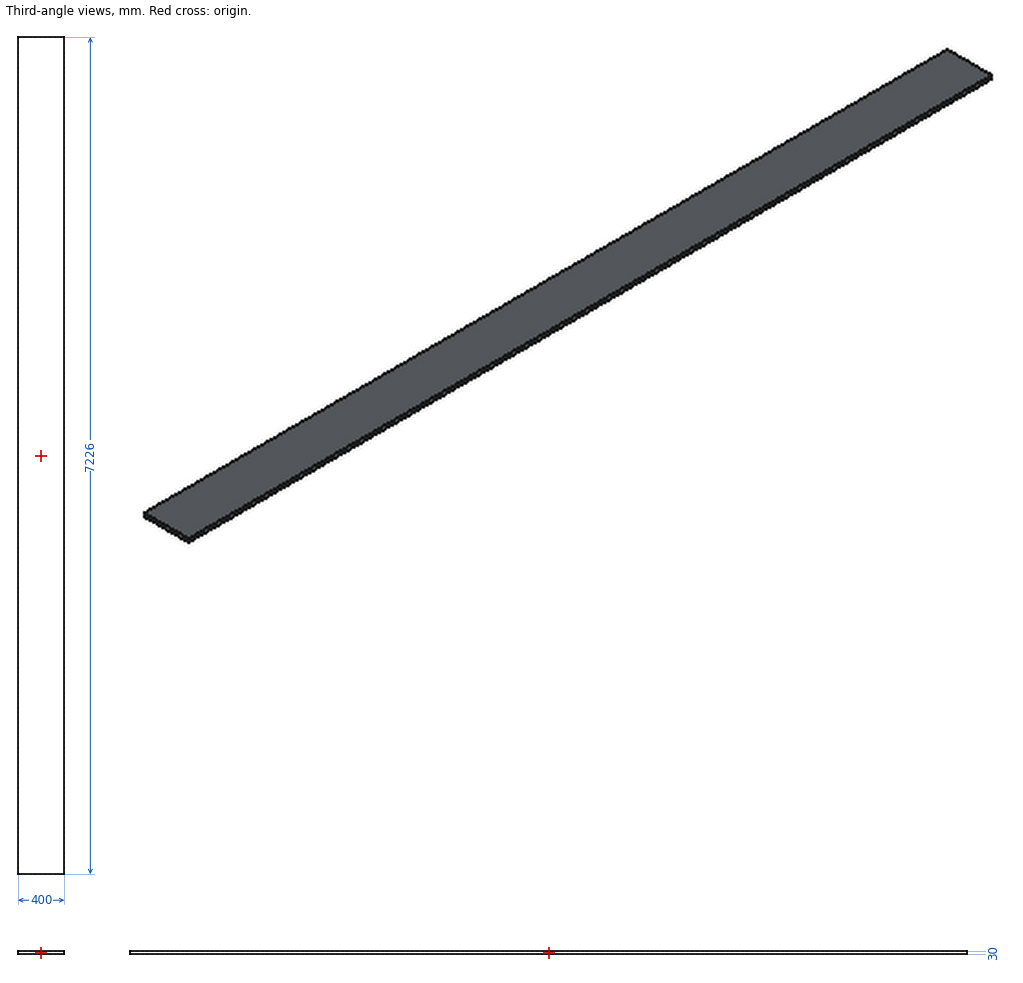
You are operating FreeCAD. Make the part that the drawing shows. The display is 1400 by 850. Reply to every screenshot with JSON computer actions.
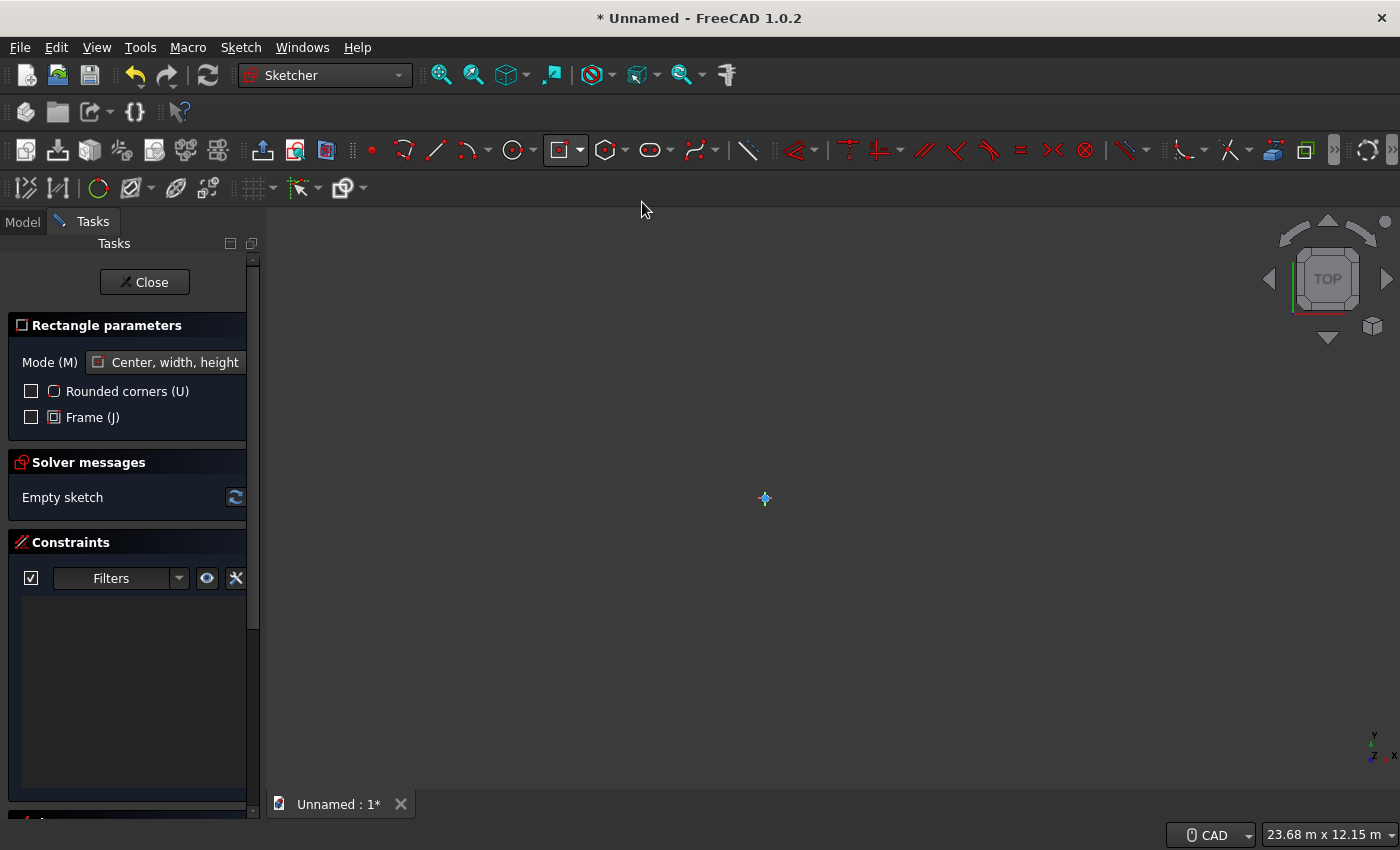
{"action": "scroll", "coordinate": [765, 498], "scroll_direction": "up", "scroll_amount": 3}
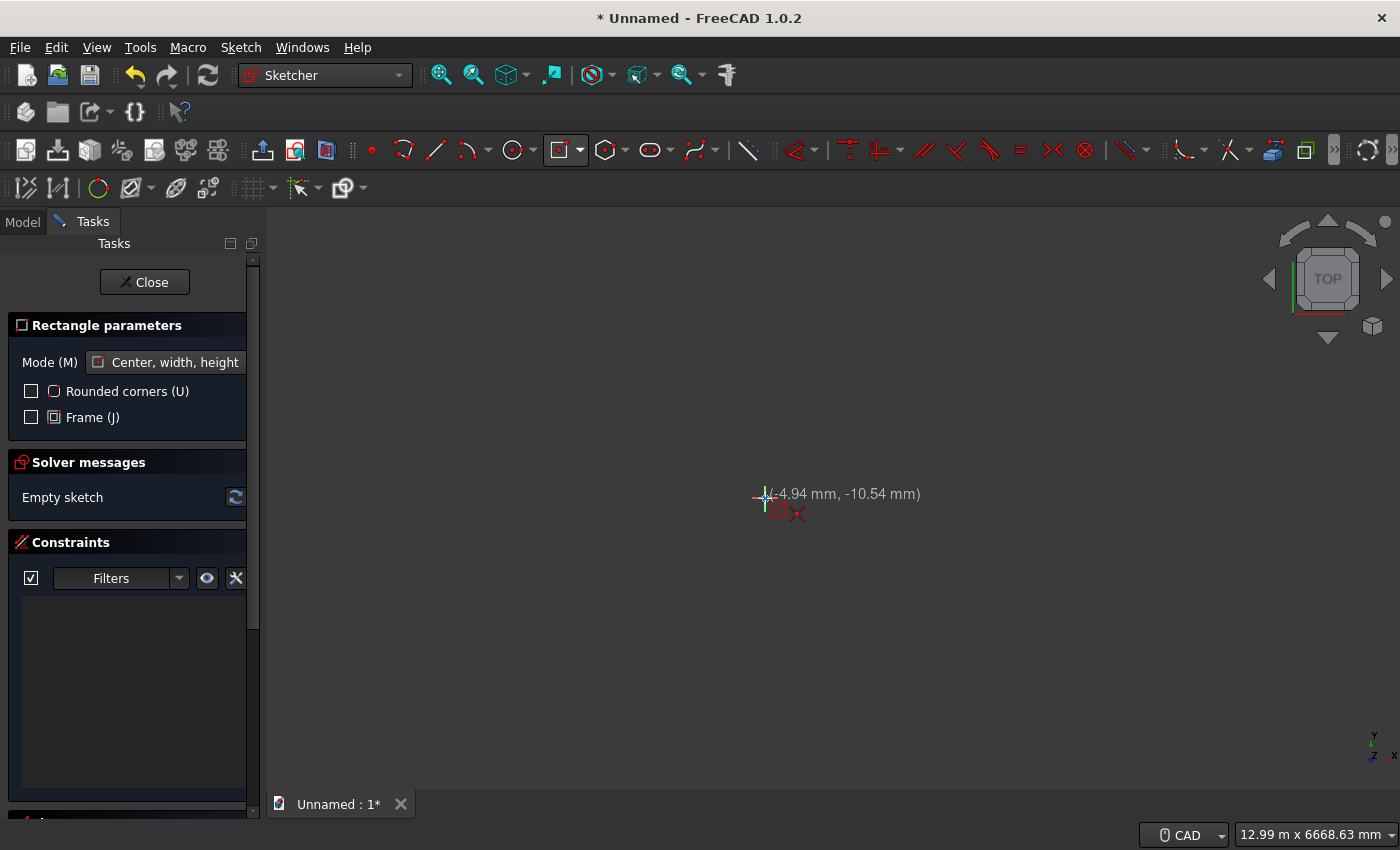
{"action": "left_click", "coordinate": [765, 498]}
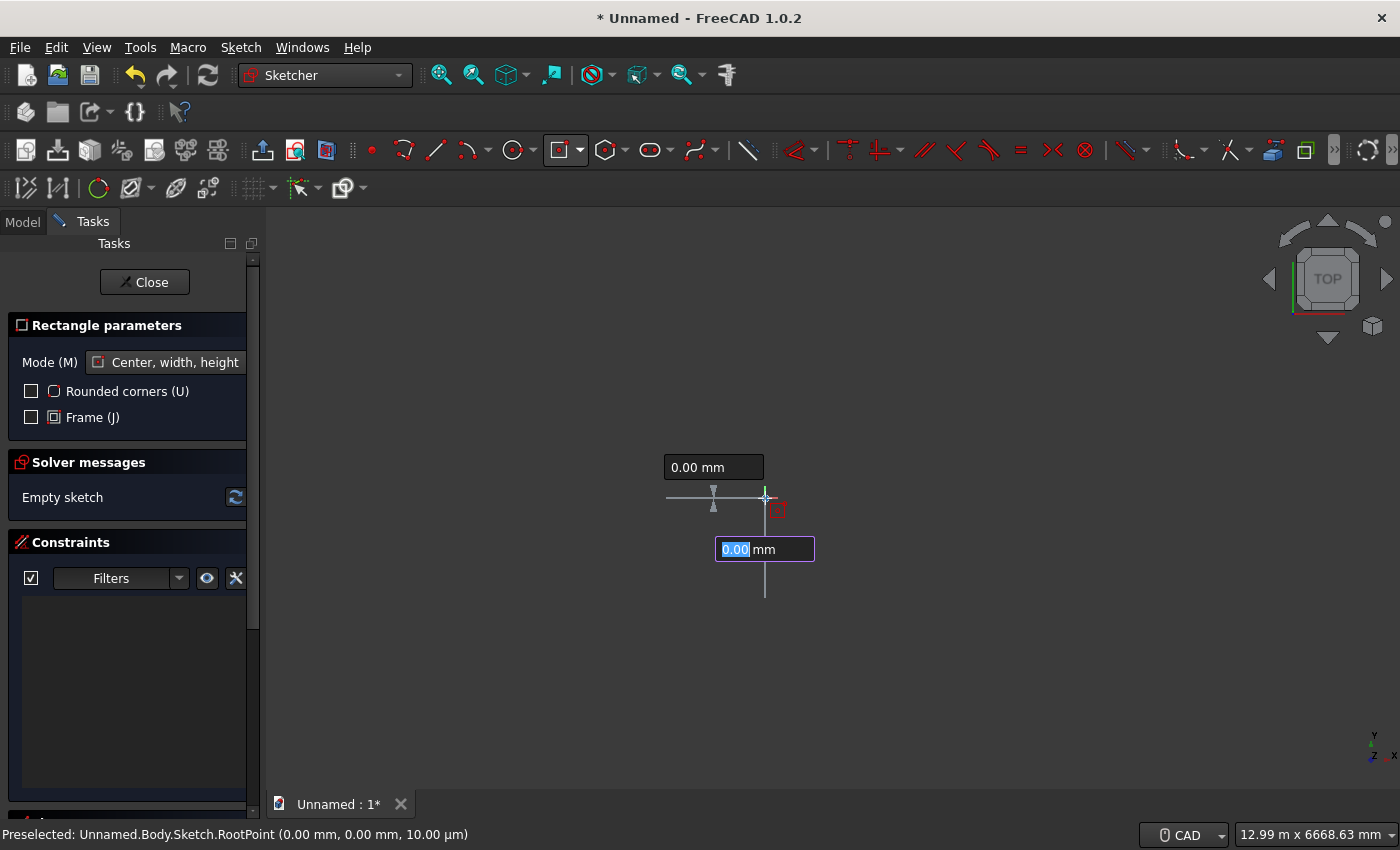
{"action": "scroll", "coordinate": [764, 497], "scroll_direction": "down", "scroll_amount": 3}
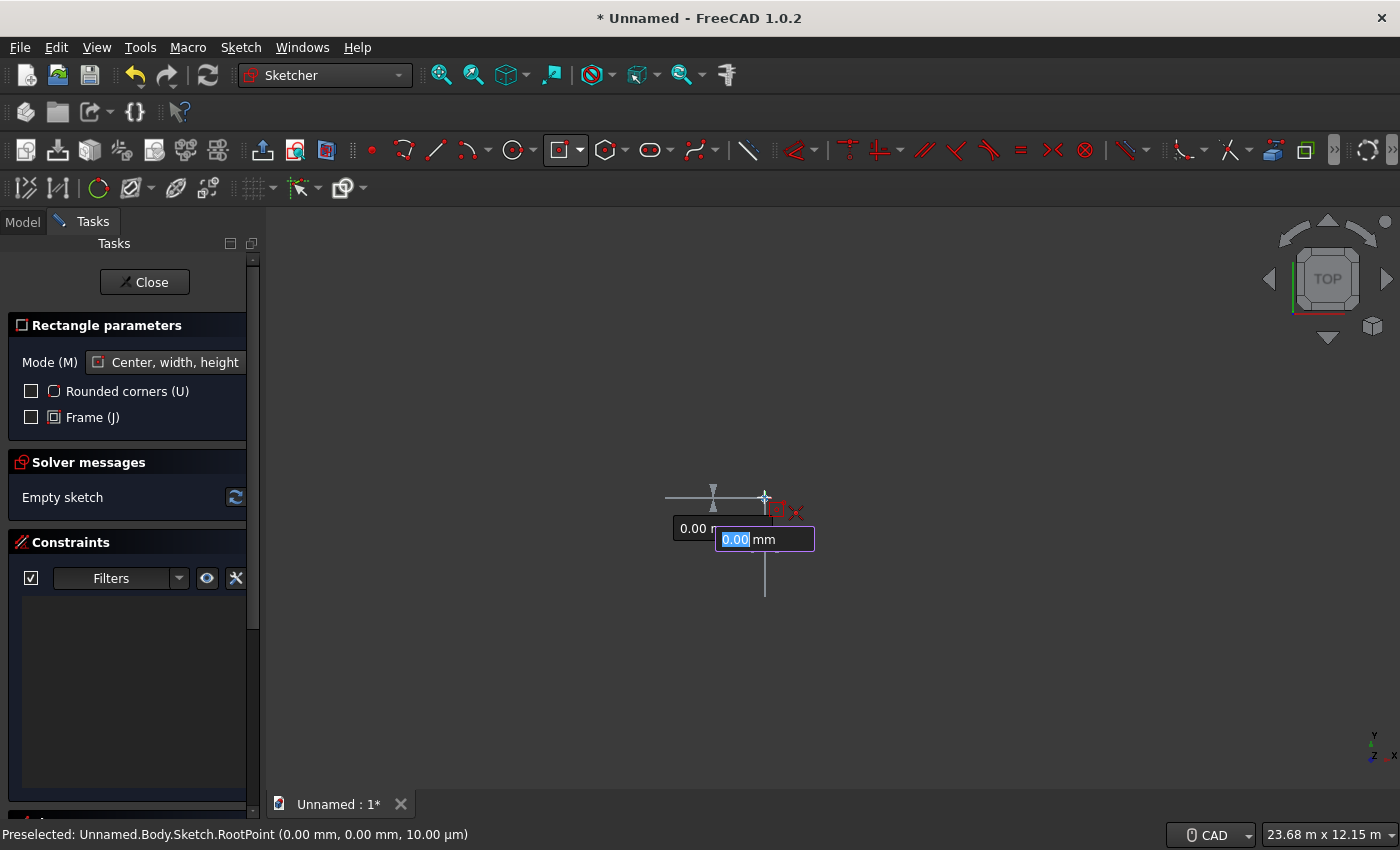
{"action": "scroll", "coordinate": [774, 325], "scroll_direction": "up", "scroll_amount": 3}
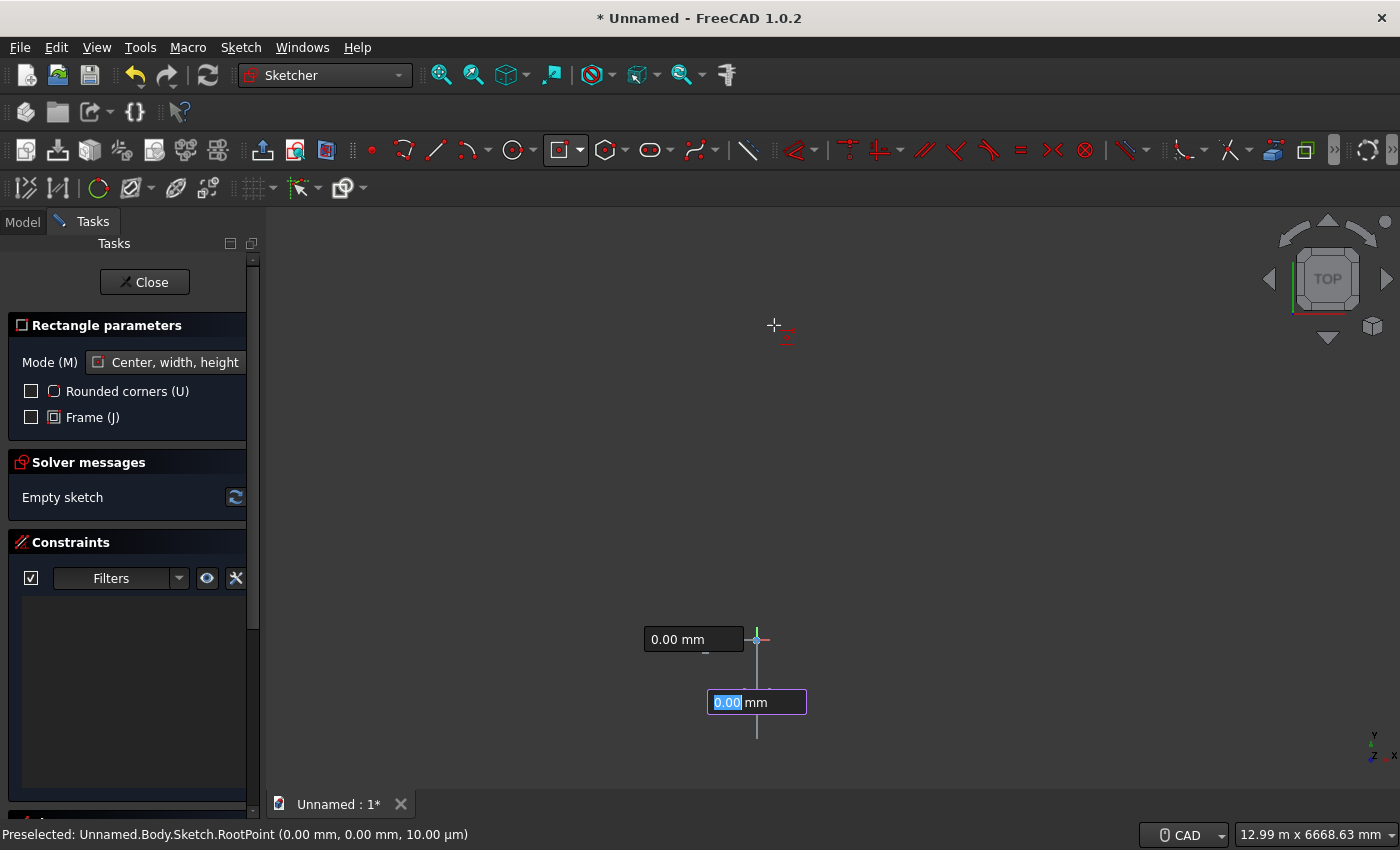
{"action": "left_click", "coordinate": [774, 325]}
{"action": "key", "text": "Escape"}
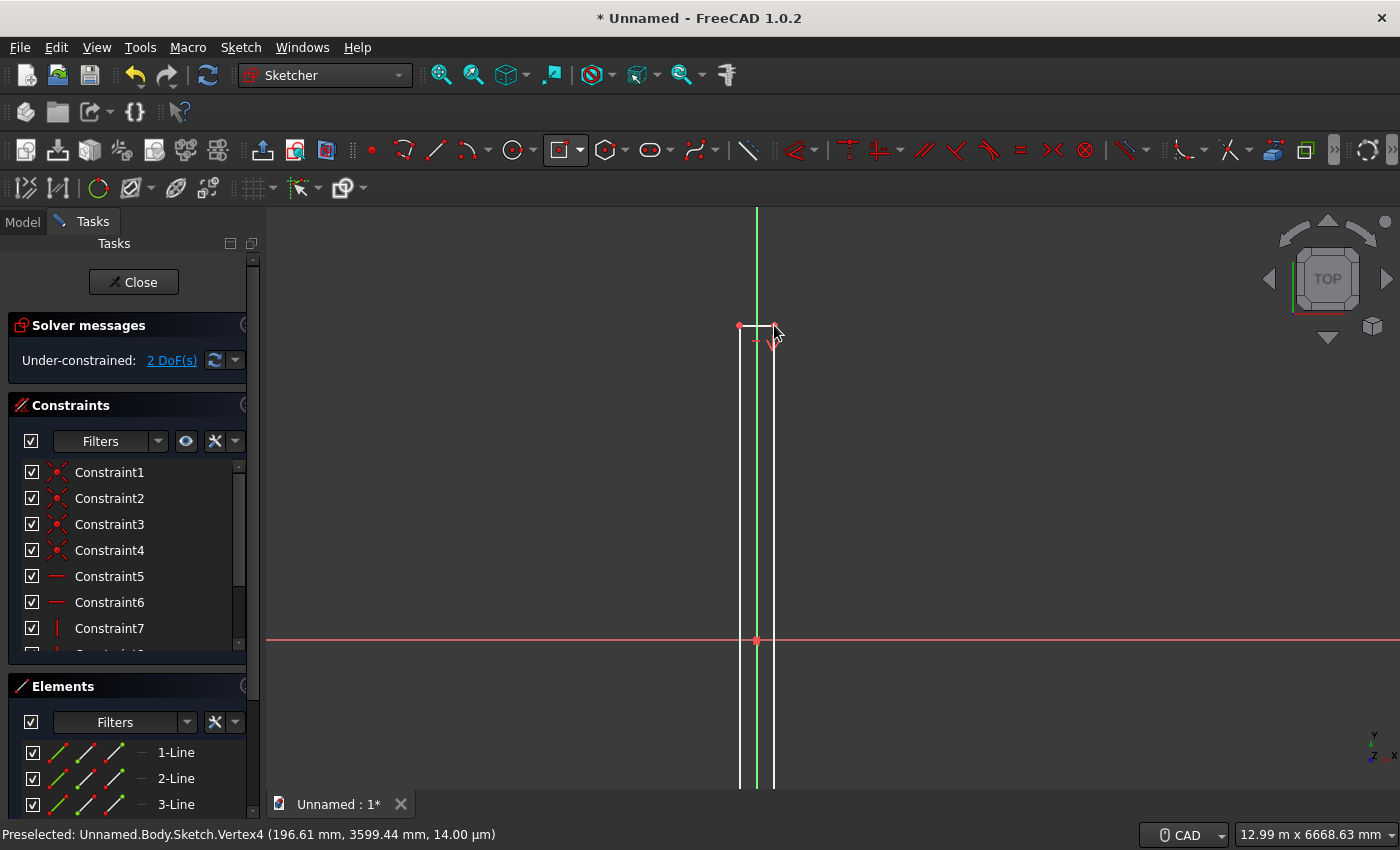
{"action": "key", "text": "d"}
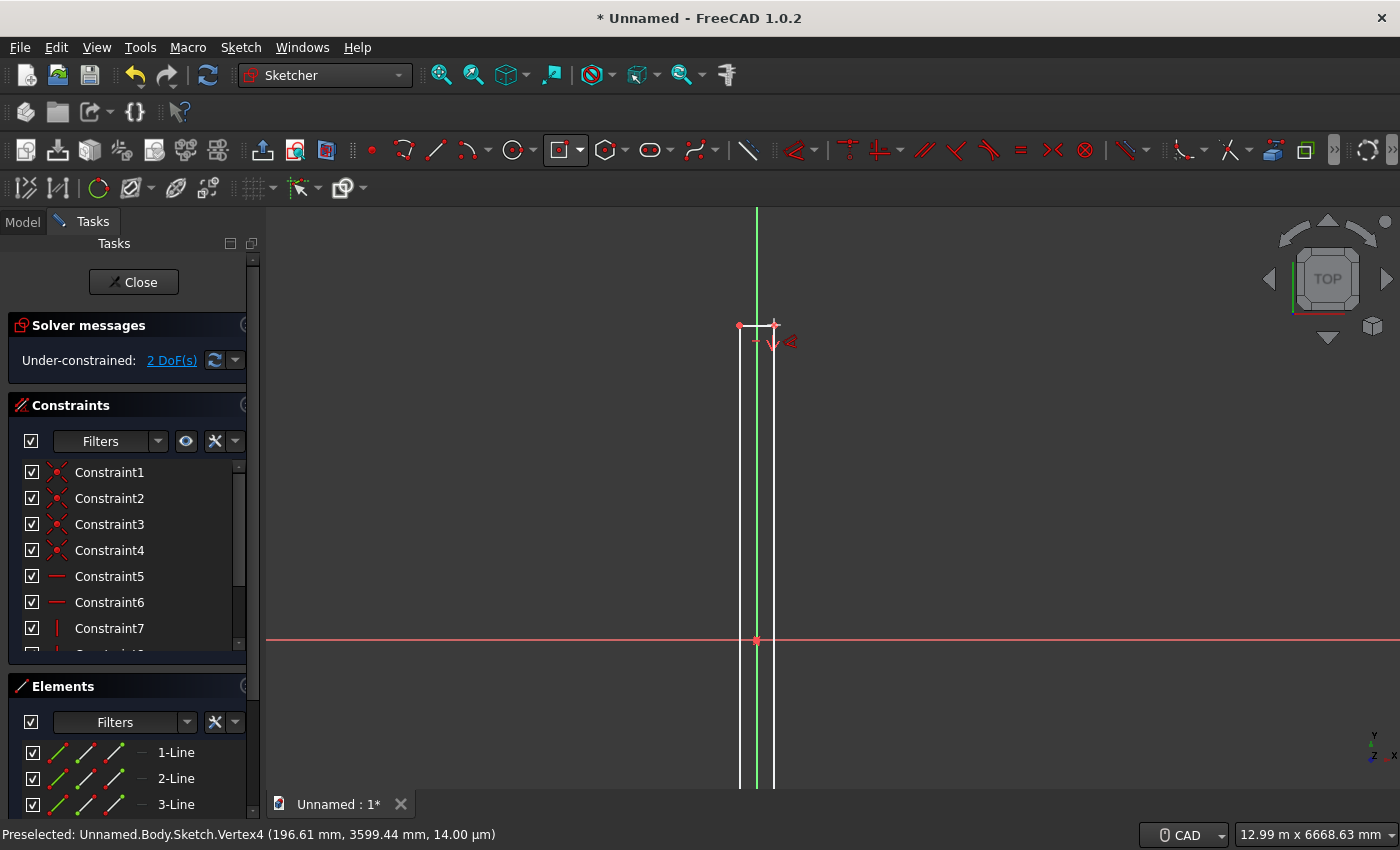
{"action": "scroll", "coordinate": [774, 325], "scroll_direction": "down", "scroll_amount": 3}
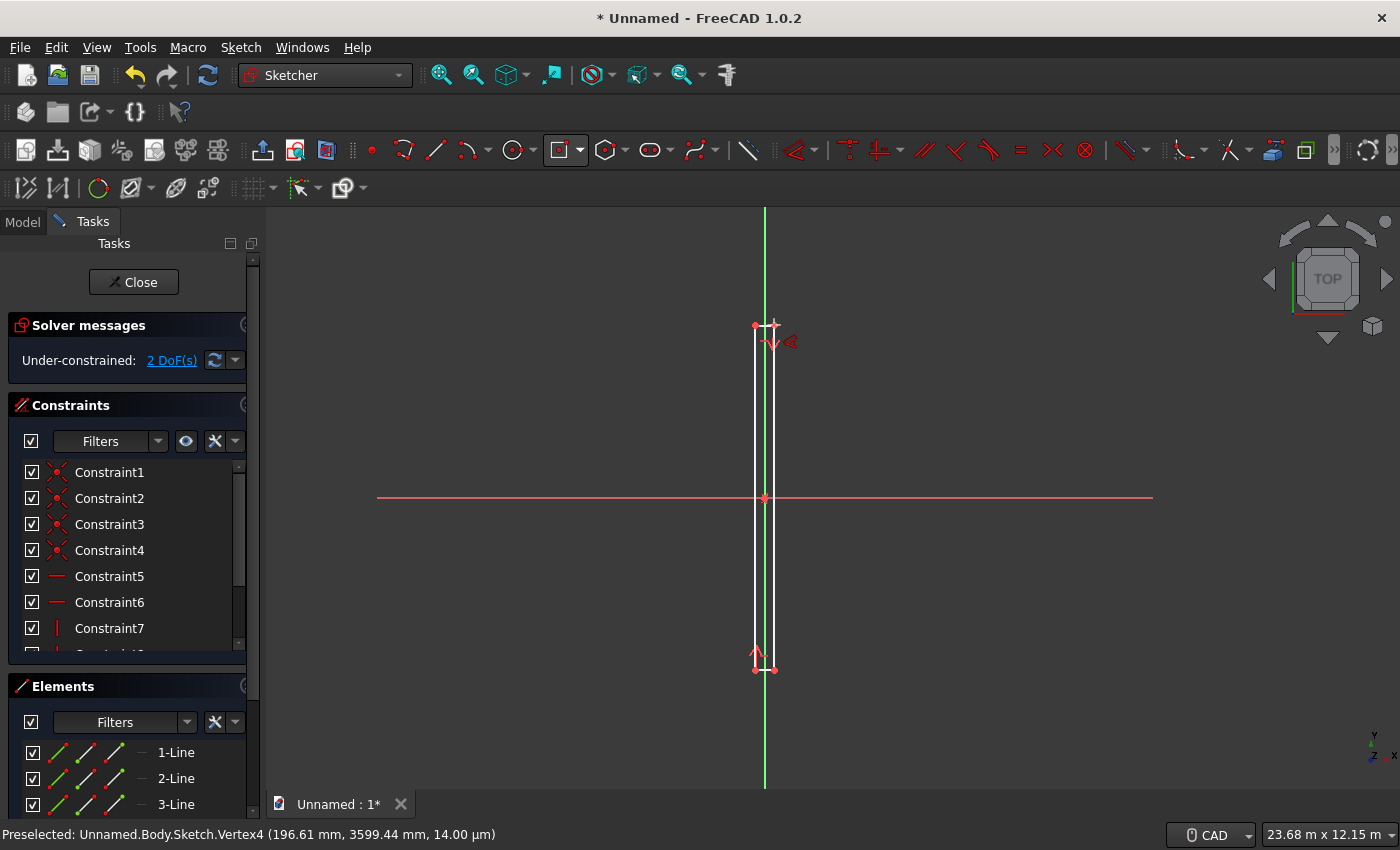
{"action": "scroll", "coordinate": [763, 670], "scroll_direction": "up", "scroll_amount": 4}